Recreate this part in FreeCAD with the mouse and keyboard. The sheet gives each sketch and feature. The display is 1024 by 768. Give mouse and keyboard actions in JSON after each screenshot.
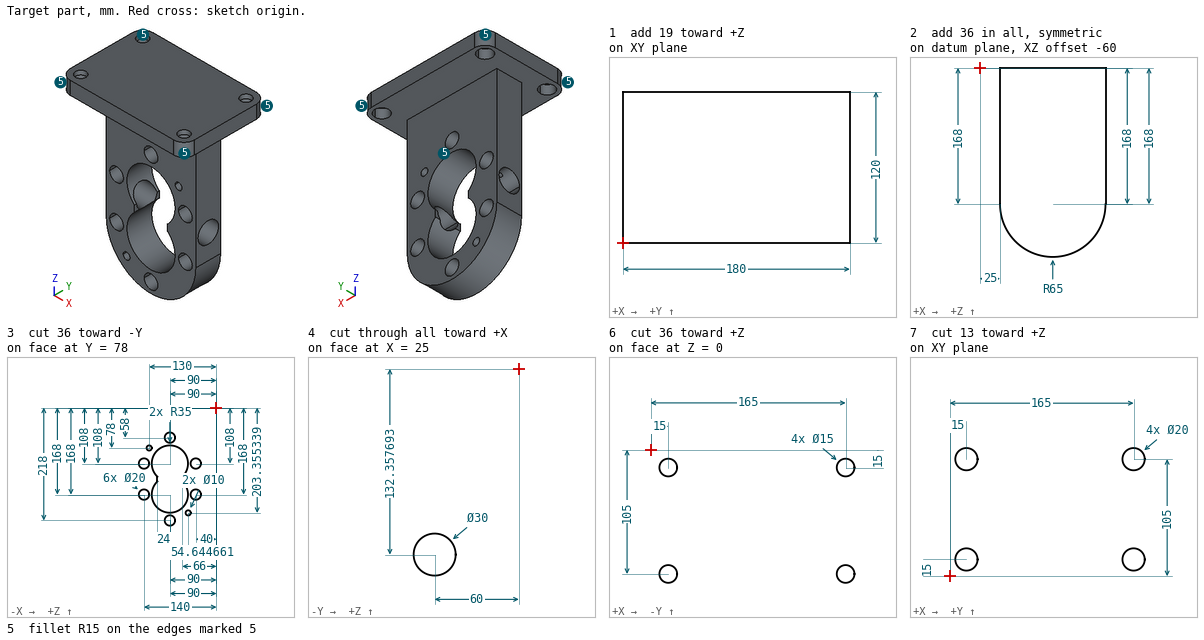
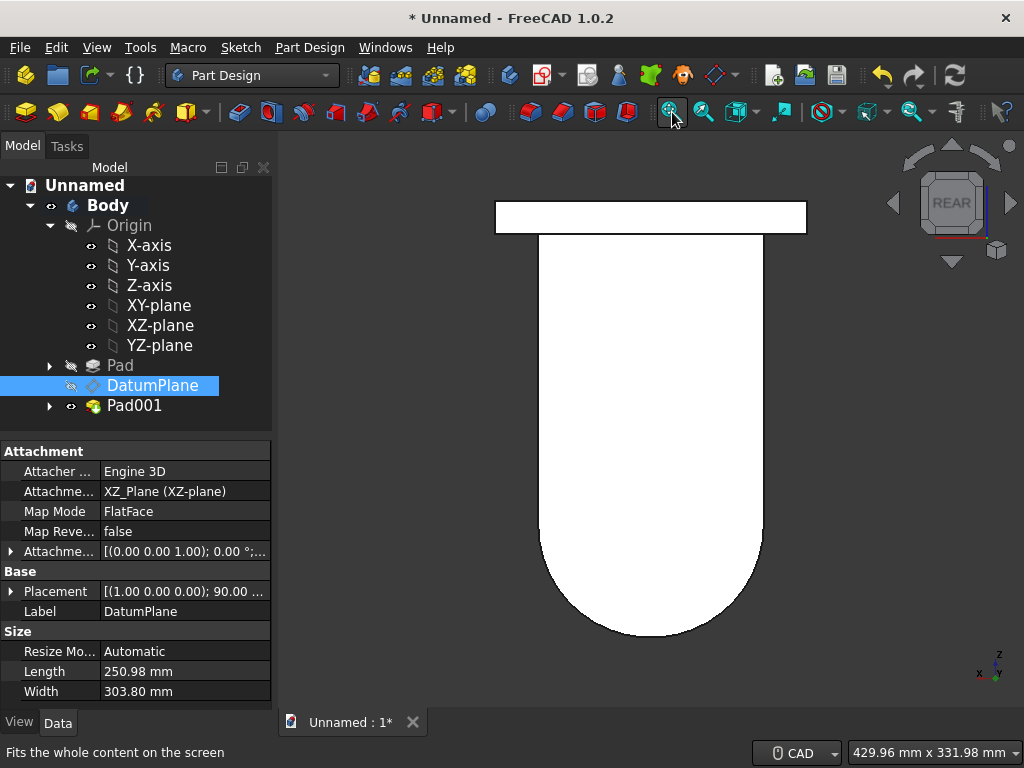
{"action": "left_click", "coordinate": [651, 377]}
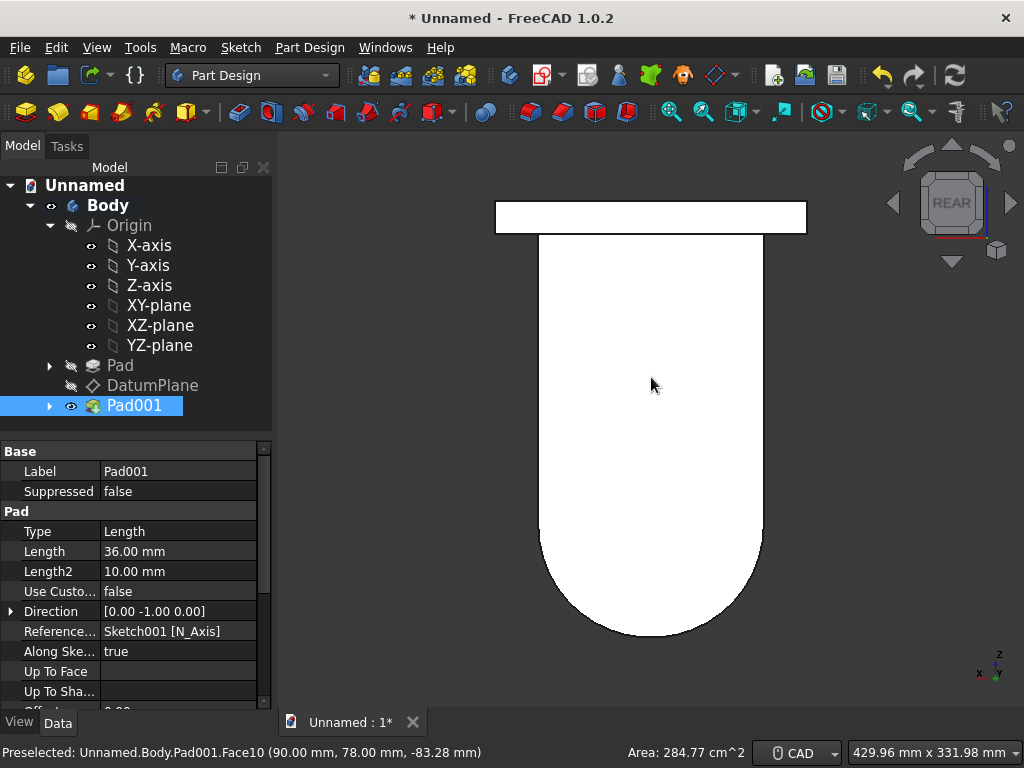
{"action": "left_click", "coordinate": [542, 76]}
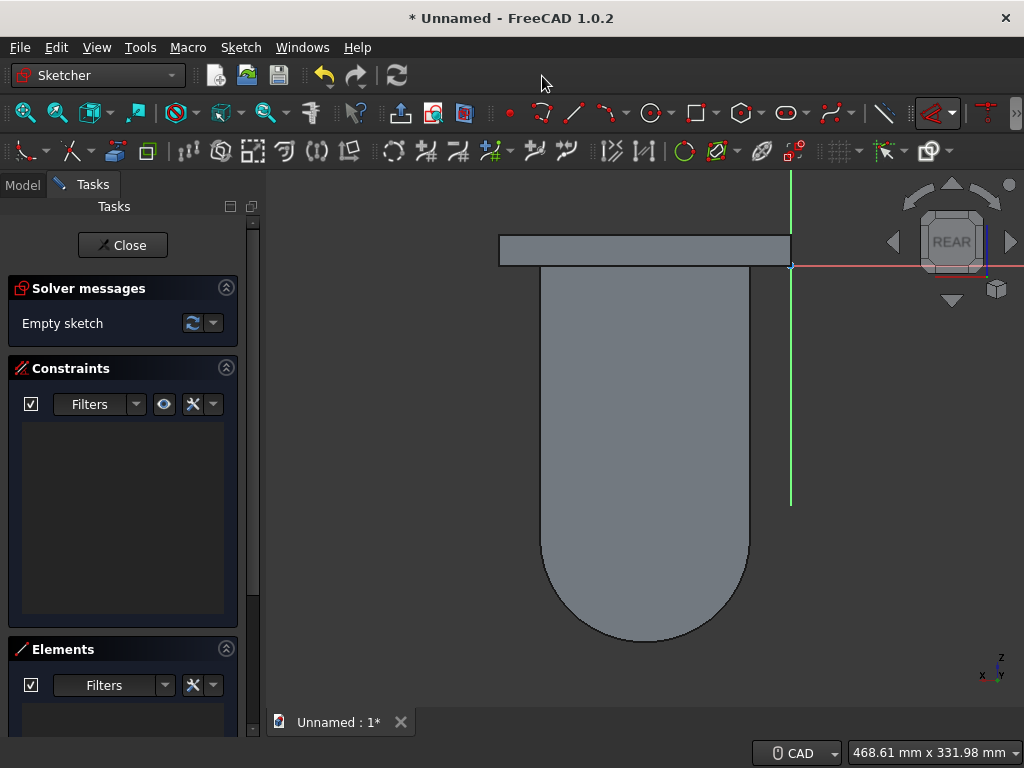
{"action": "left_click", "coordinate": [466, 114]}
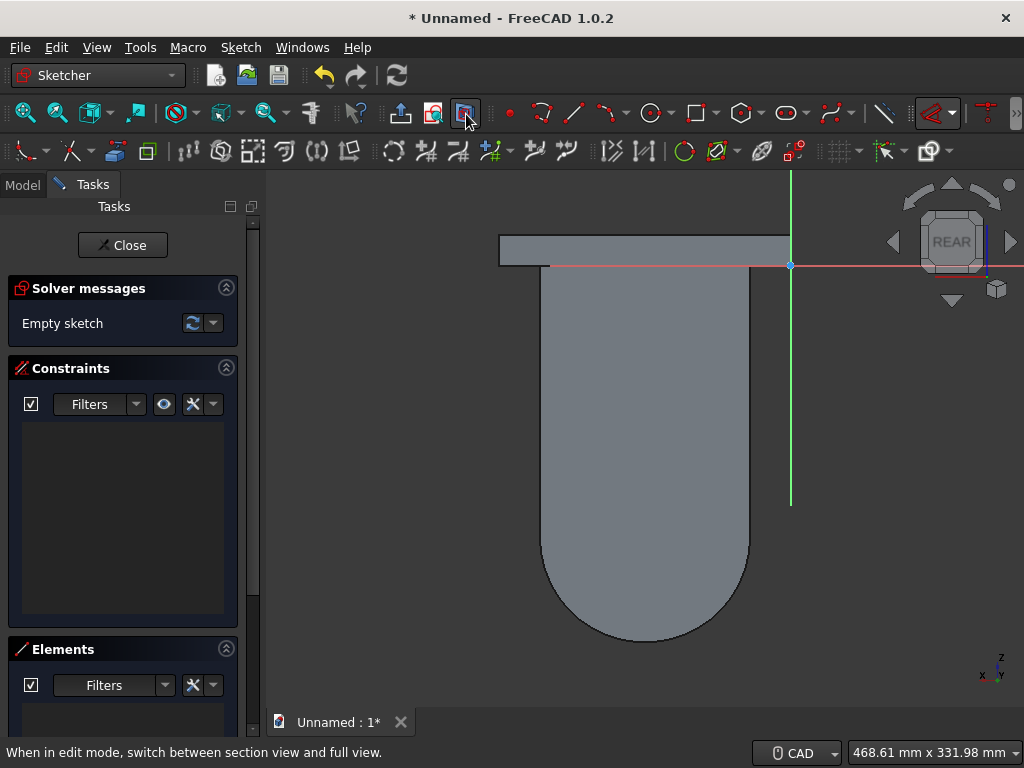
{"action": "left_click", "coordinate": [574, 114]}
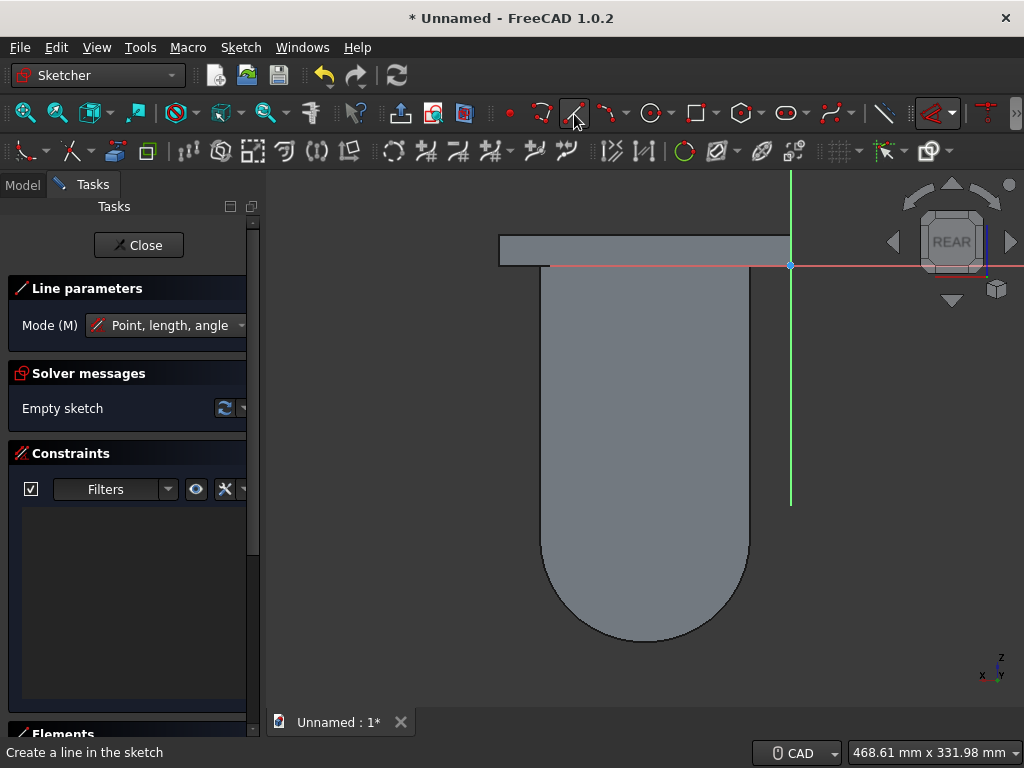
{"action": "left_click", "coordinate": [684, 496]}
{"action": "left_click", "coordinate": [684, 481]}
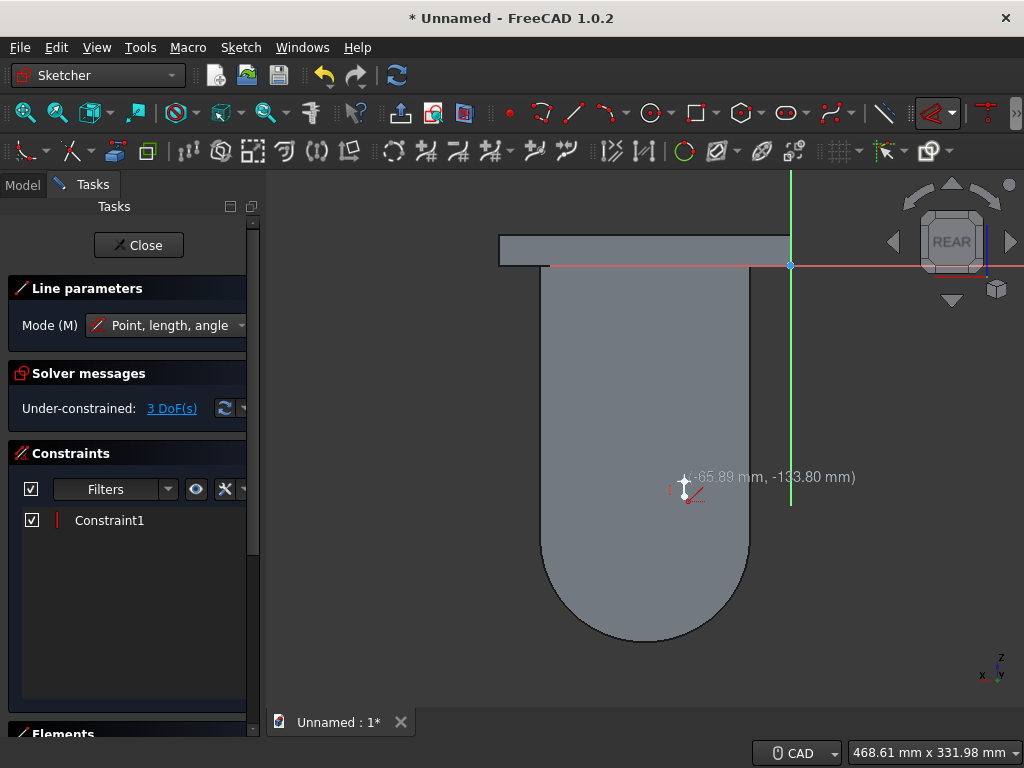
{"action": "left_click", "coordinate": [606, 481]}
{"action": "left_click", "coordinate": [606, 496]}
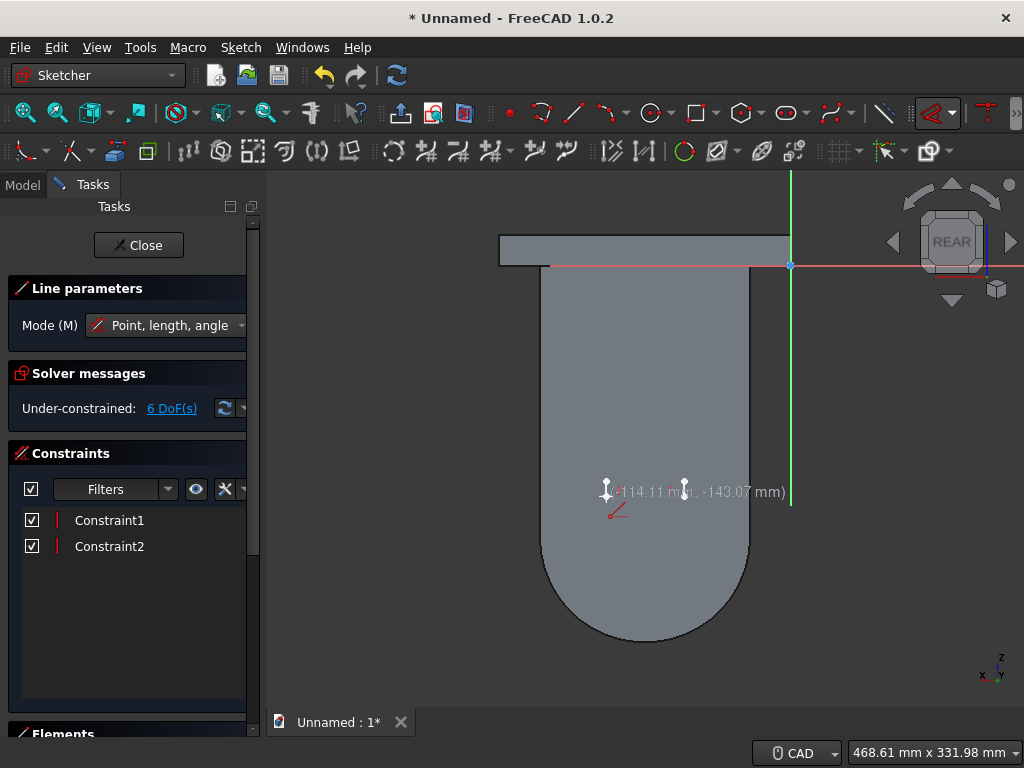
{"action": "left_click", "coordinate": [606, 114]}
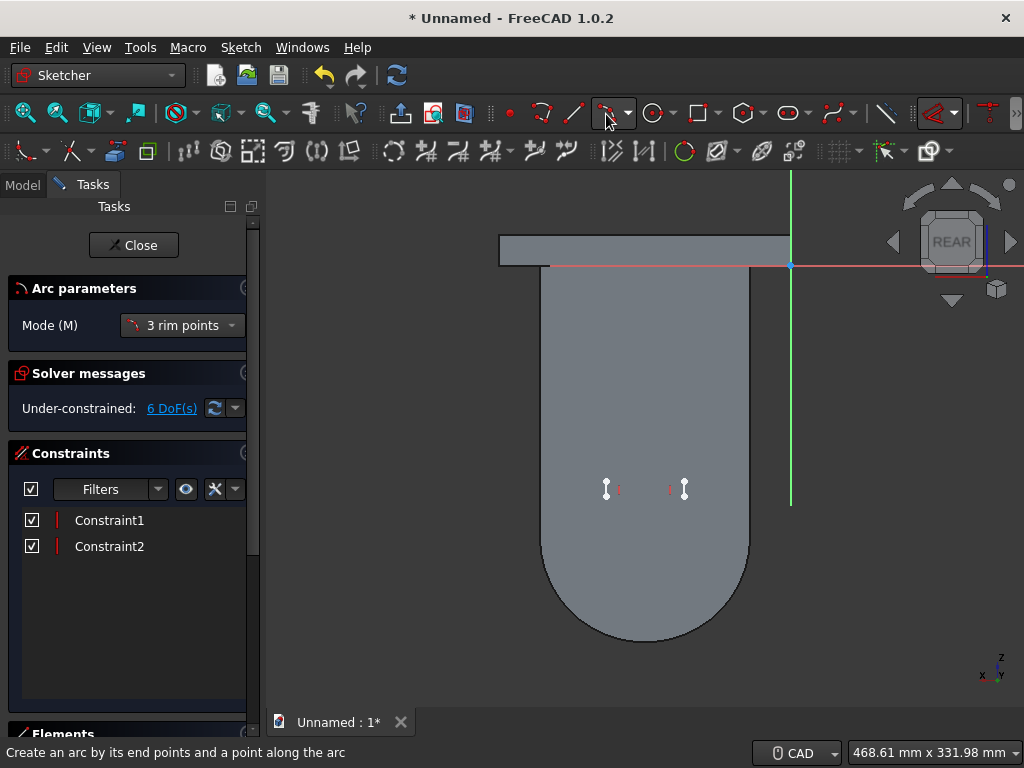
{"action": "scroll", "coordinate": [684, 481], "scroll_direction": "up", "scroll_amount": 4}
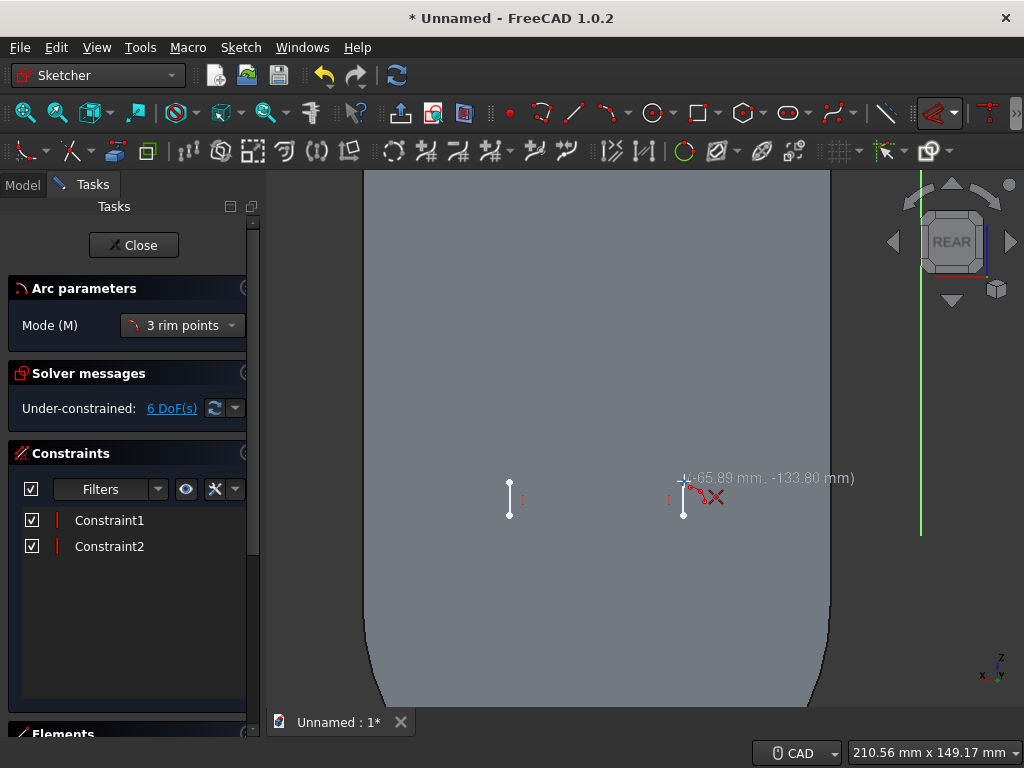
{"action": "left_click", "coordinate": [683, 483]}
{"action": "left_click", "coordinate": [510, 483]}
{"action": "left_click", "coordinate": [597, 264]}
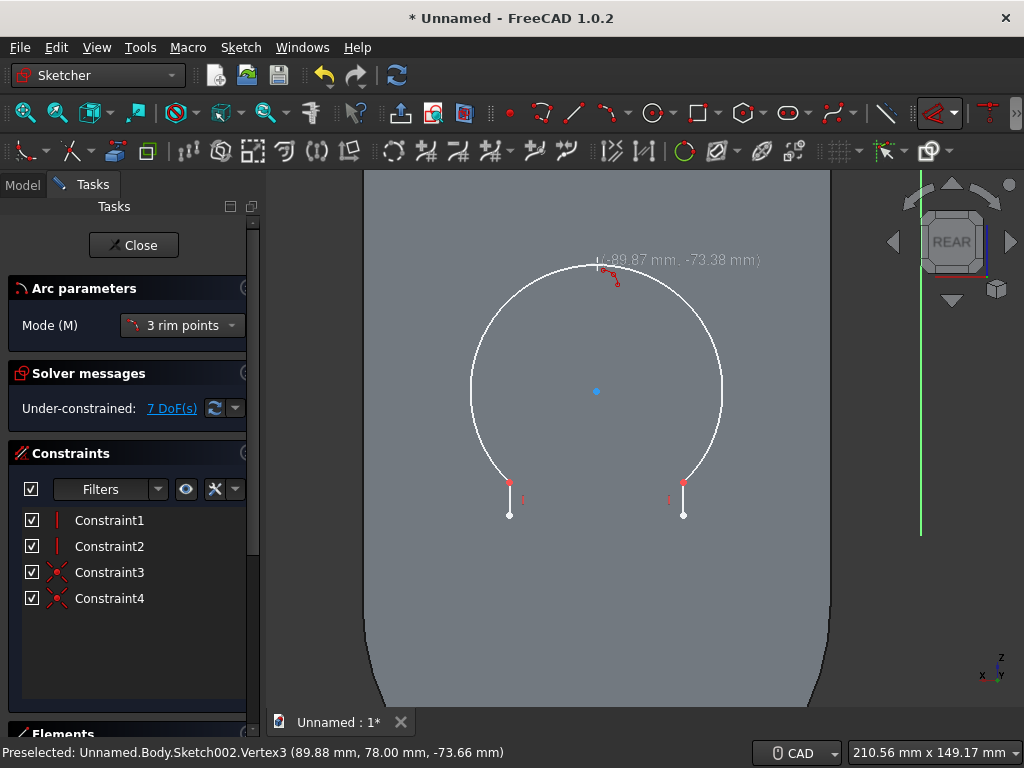
{"action": "left_click", "coordinate": [510, 516]}
{"action": "left_click", "coordinate": [683, 516]}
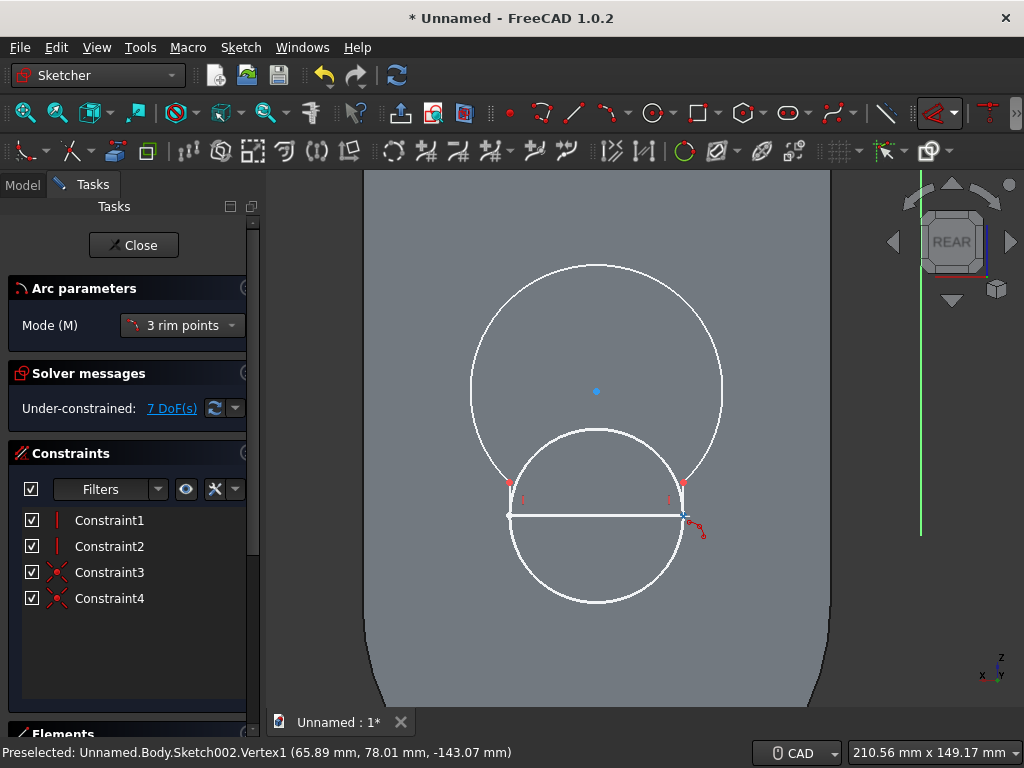
{"action": "scroll", "coordinate": [516, 461], "scroll_direction": "down", "scroll_amount": 4}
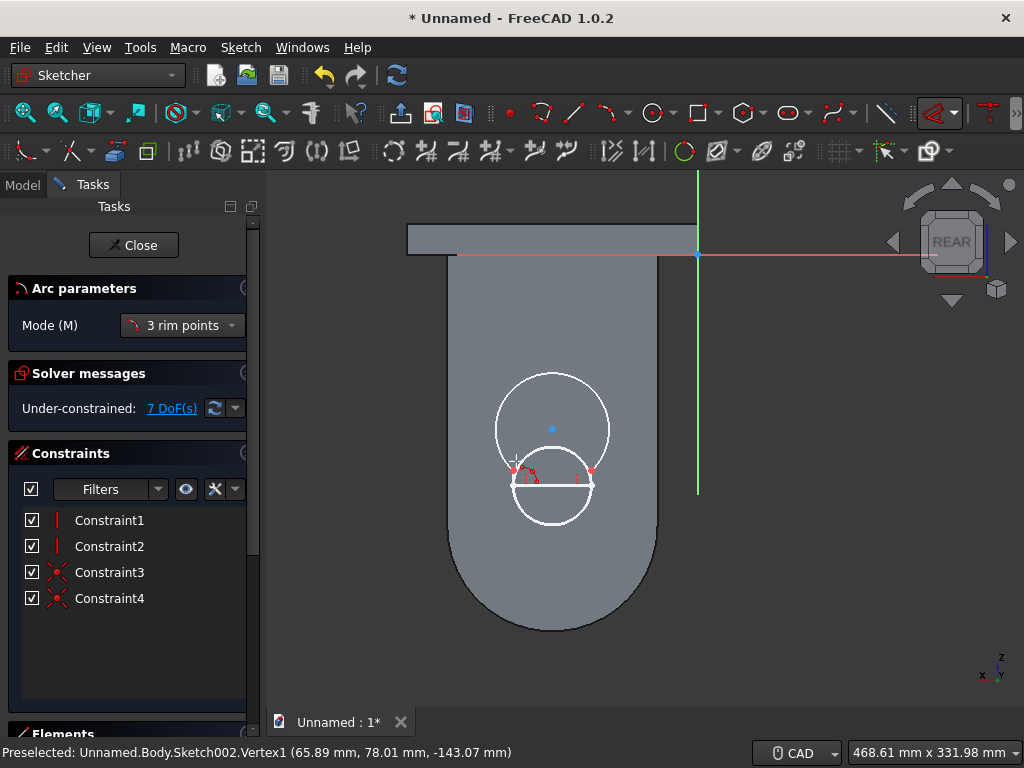
{"action": "left_click", "coordinate": [552, 583]}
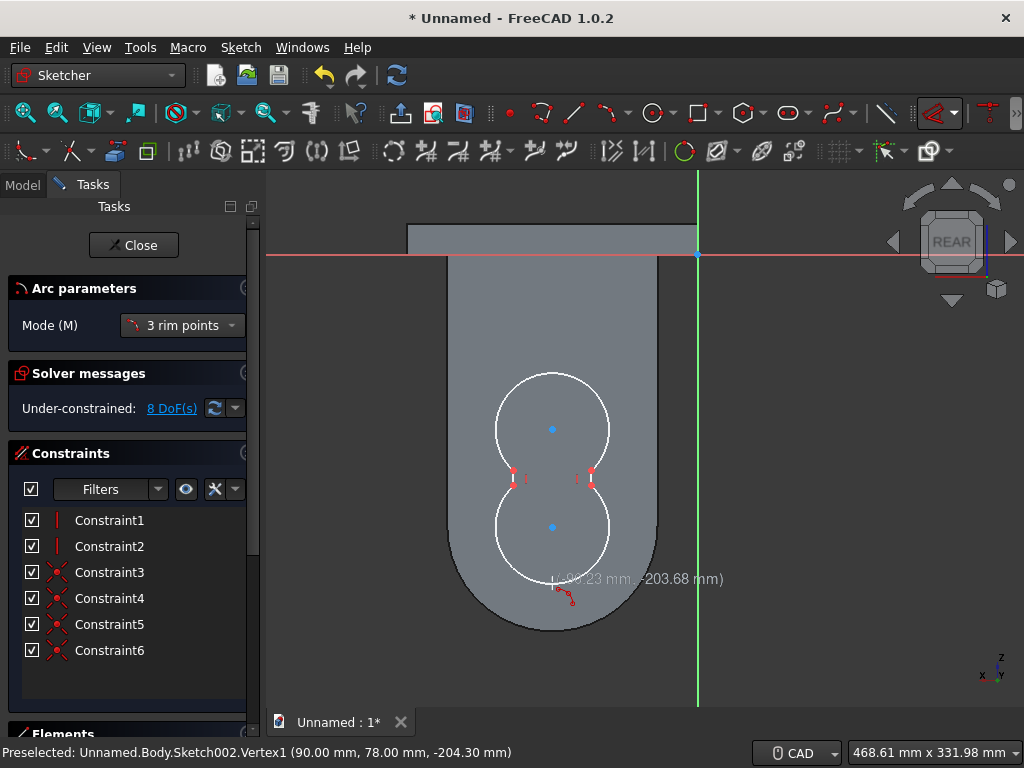
{"action": "left_click", "coordinate": [654, 114]}